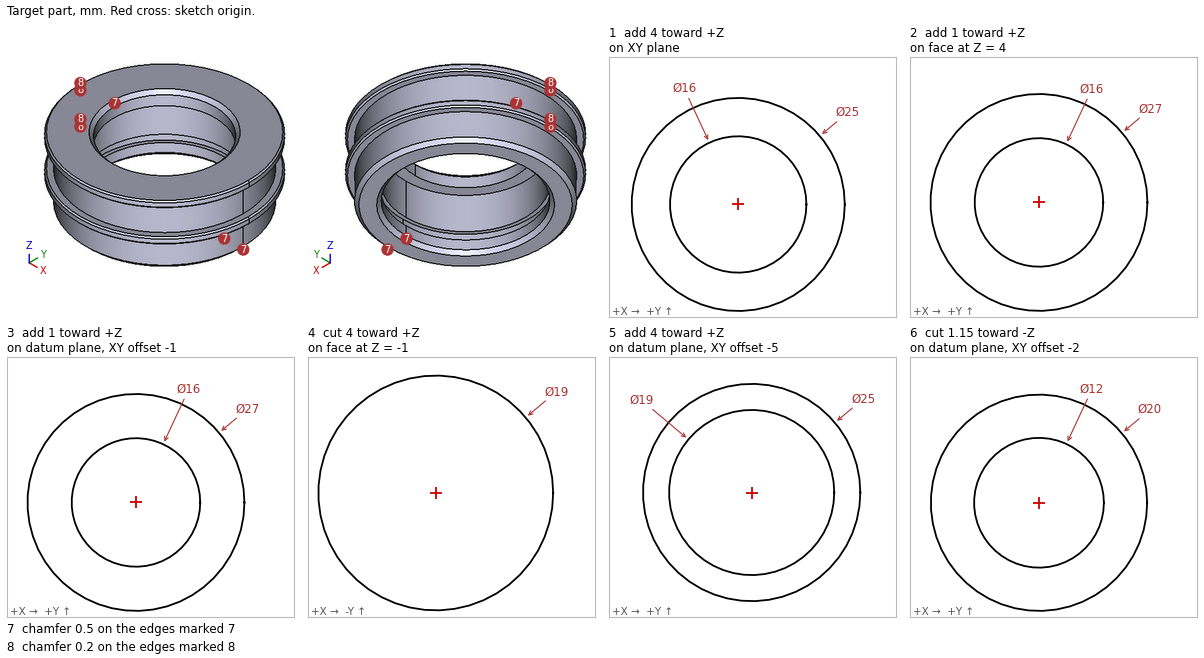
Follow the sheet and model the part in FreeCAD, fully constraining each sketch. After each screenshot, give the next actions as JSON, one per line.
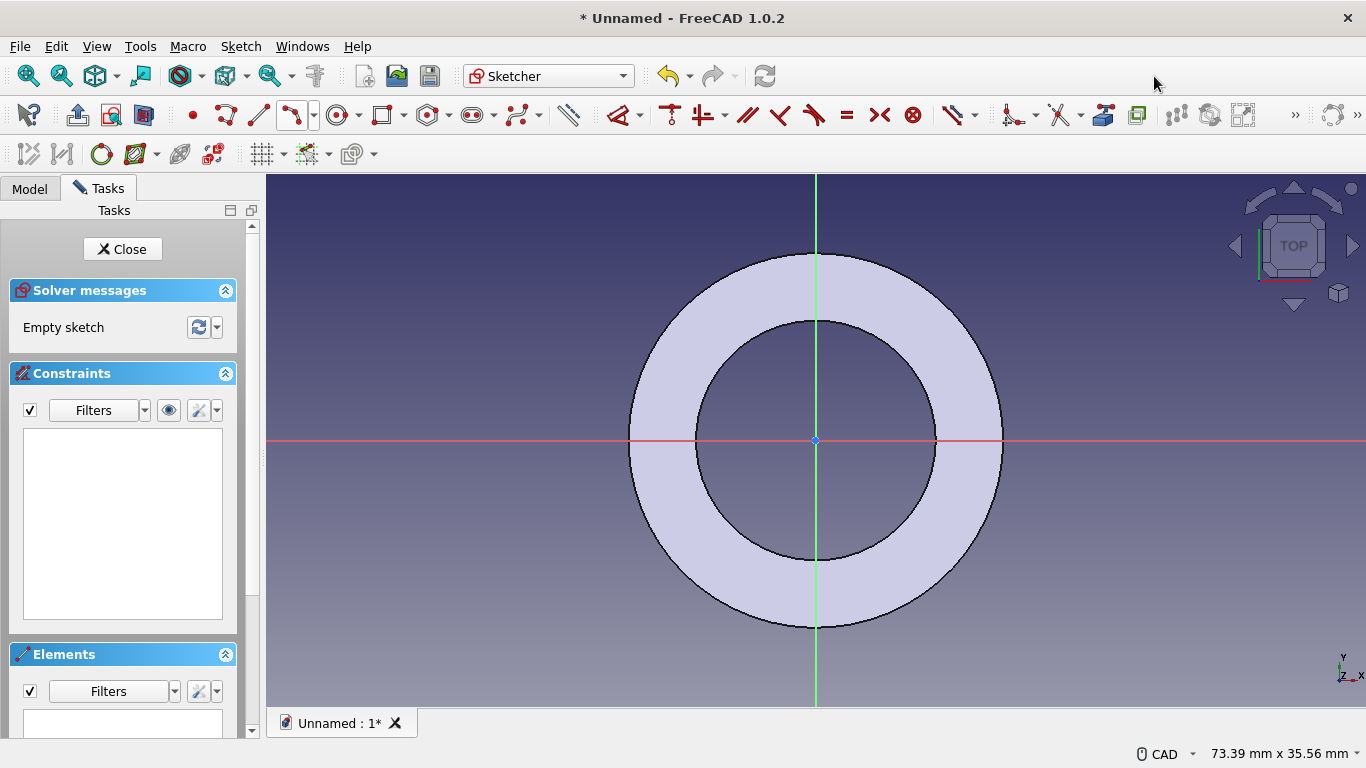
{"action": "left_click", "coordinate": [336, 116]}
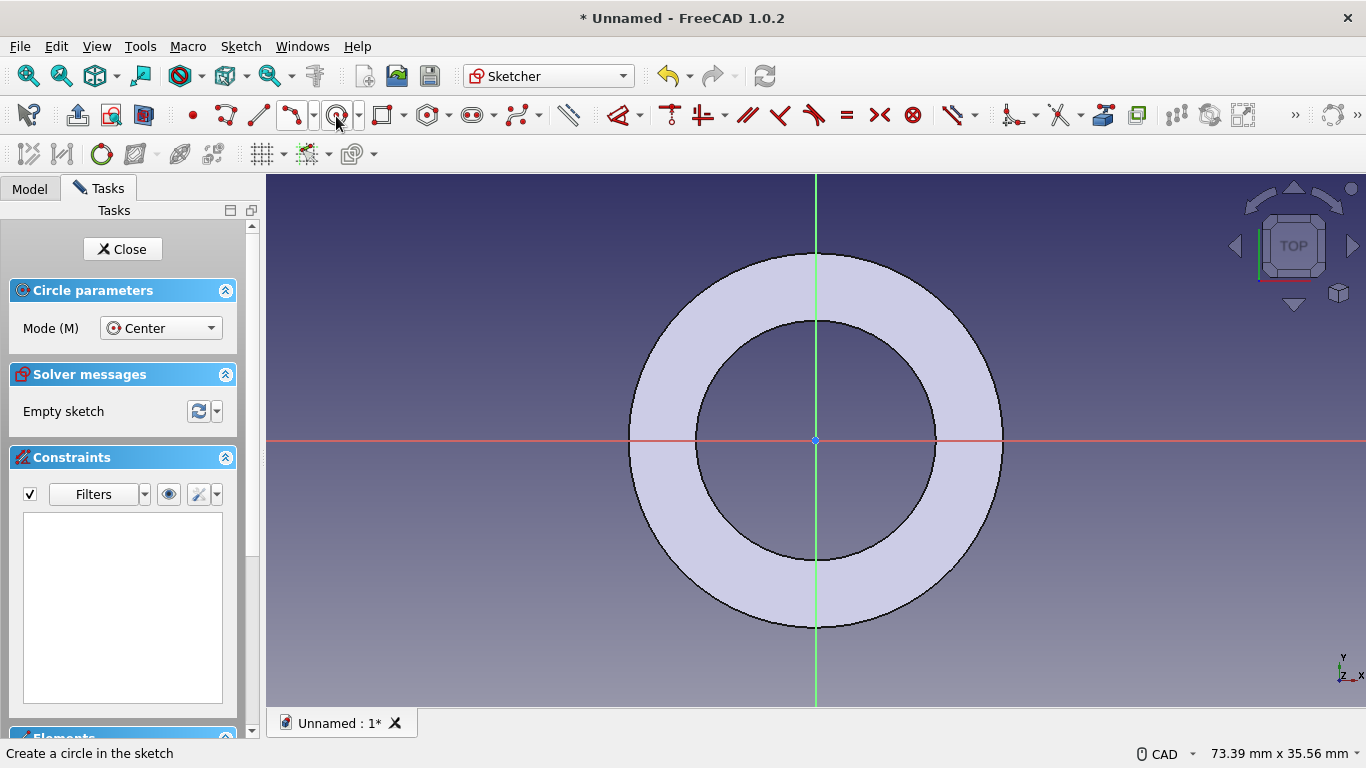
{"action": "left_click", "coordinate": [816, 440]}
{"action": "left_click", "coordinate": [959, 297]}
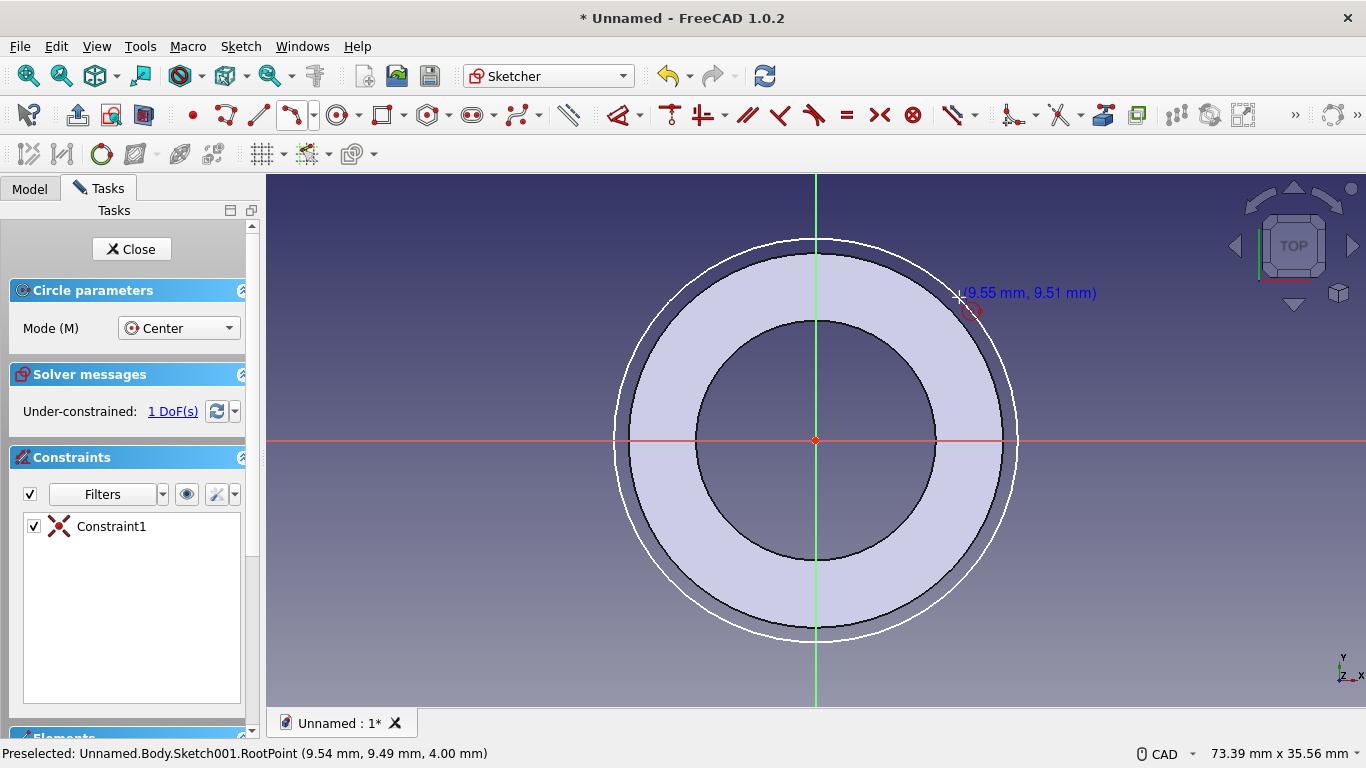
{"action": "left_click", "coordinate": [816, 440]}
{"action": "left_click", "coordinate": [901, 356]}
{"action": "key", "text": "Escape"}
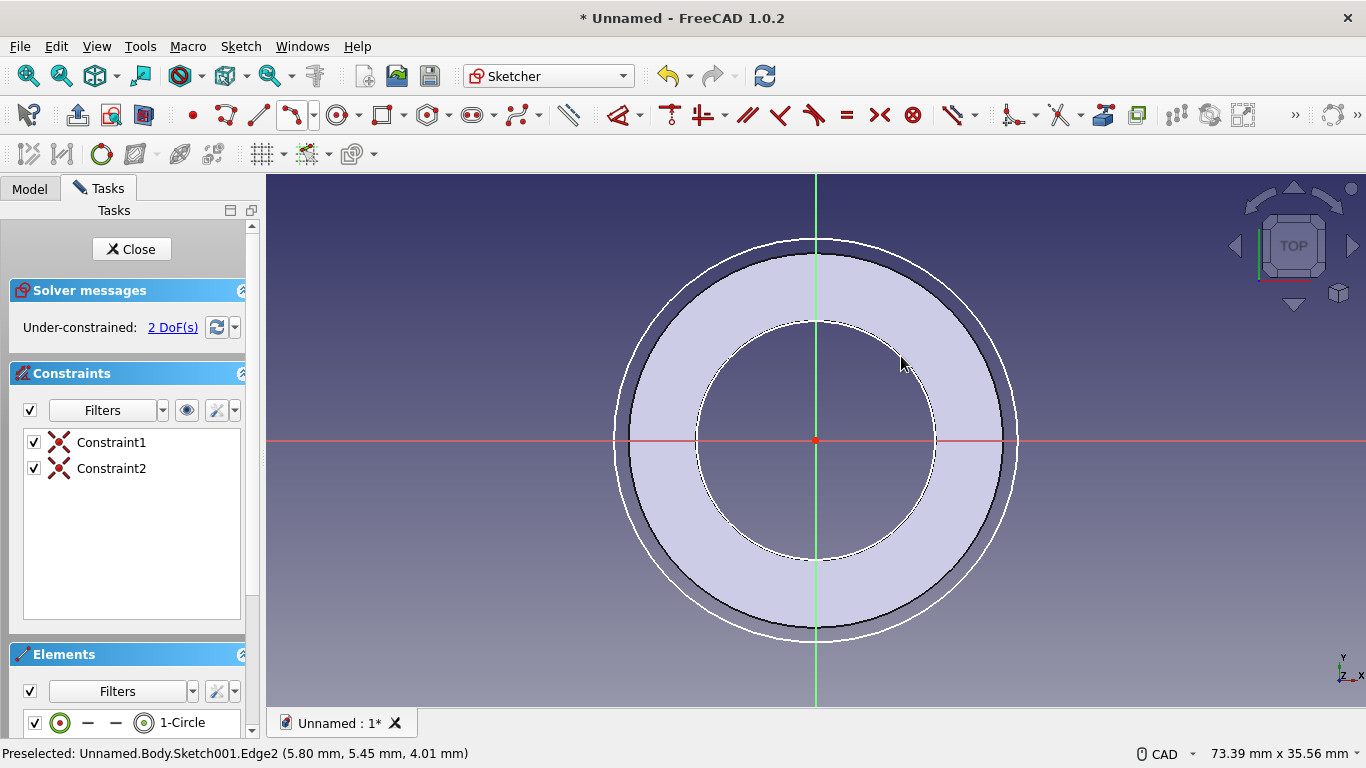
{"action": "left_click", "coordinate": [618, 116]}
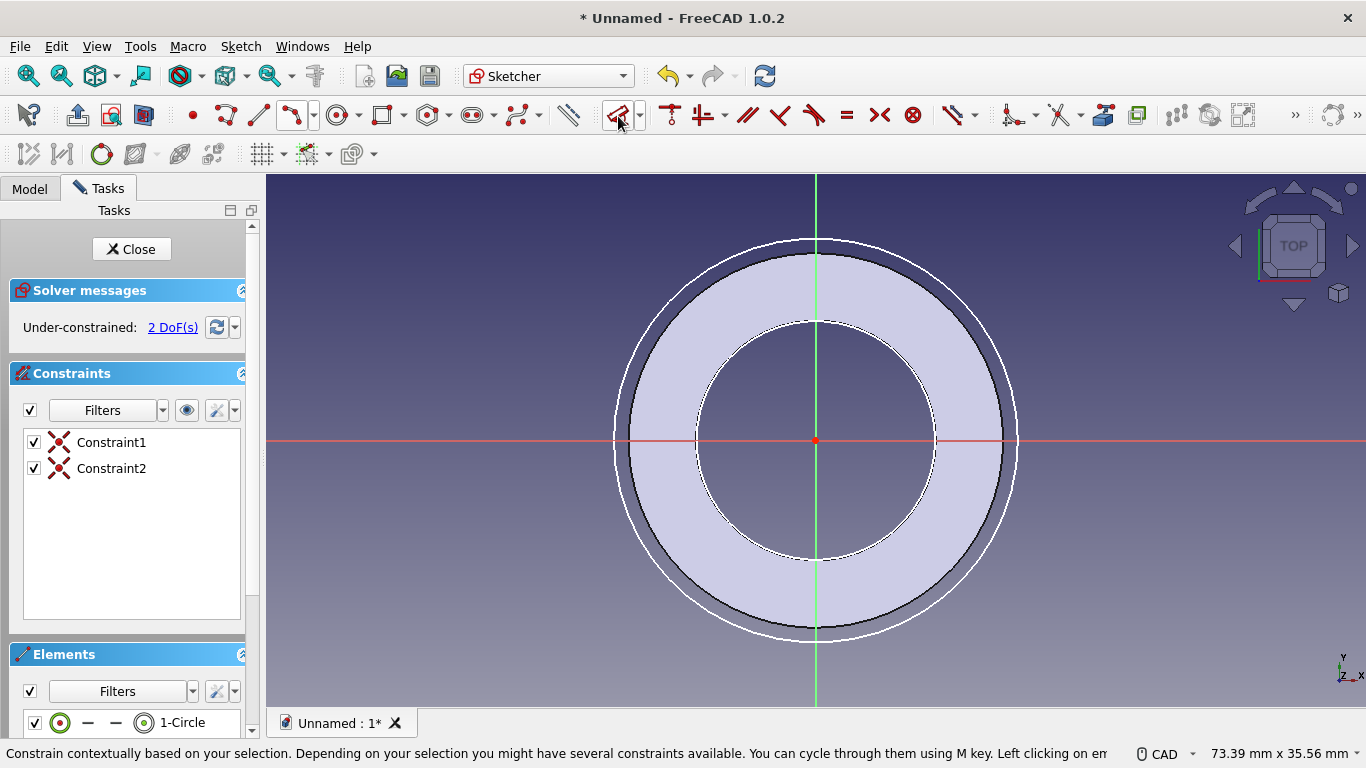
{"action": "left_click", "coordinate": [958, 297]}
{"action": "left_click", "coordinate": [981, 274]}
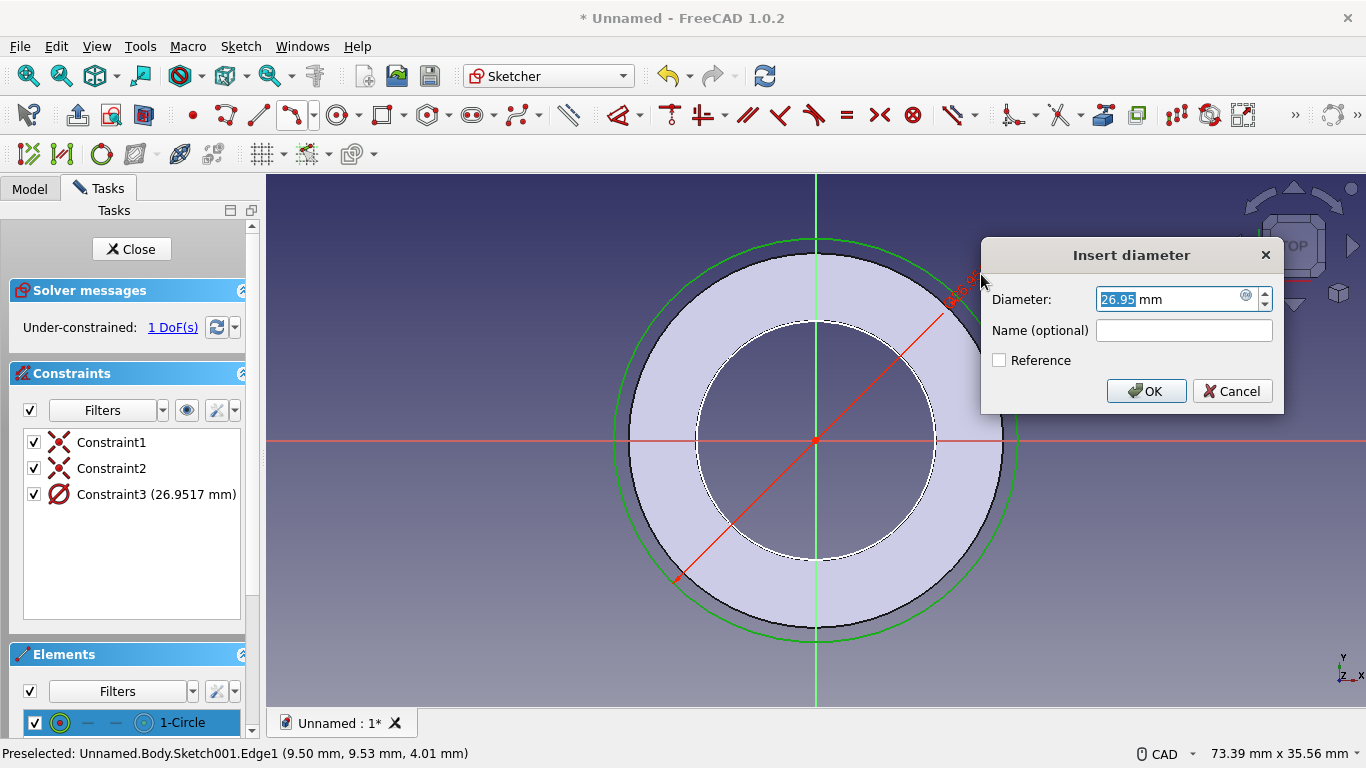
{"action": "type", "text": "27"}
{"action": "key", "text": "Return"}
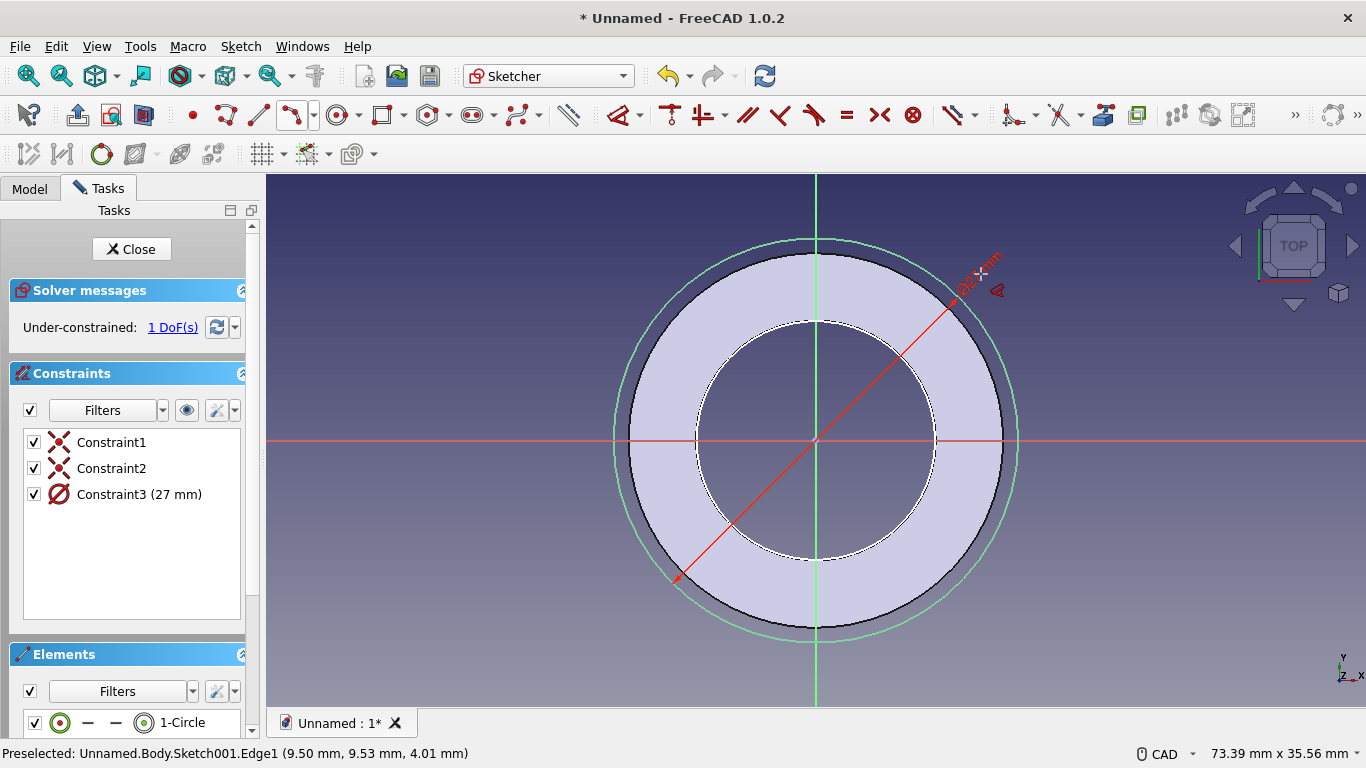
{"action": "left_click", "coordinate": [900, 356]}
{"action": "left_click", "coordinate": [923, 333]}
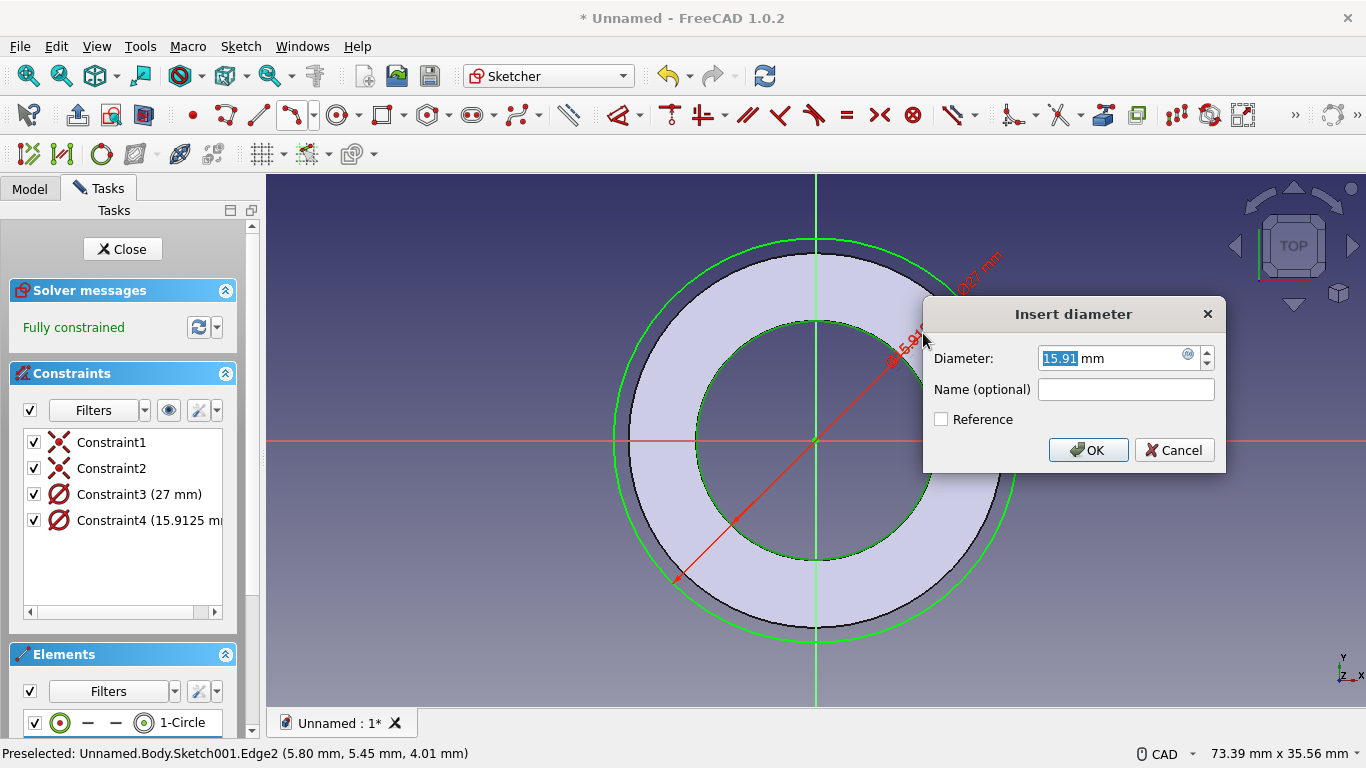
{"action": "type", "text": "16"}
{"action": "key", "text": "Return"}
{"action": "key", "text": "Escape"}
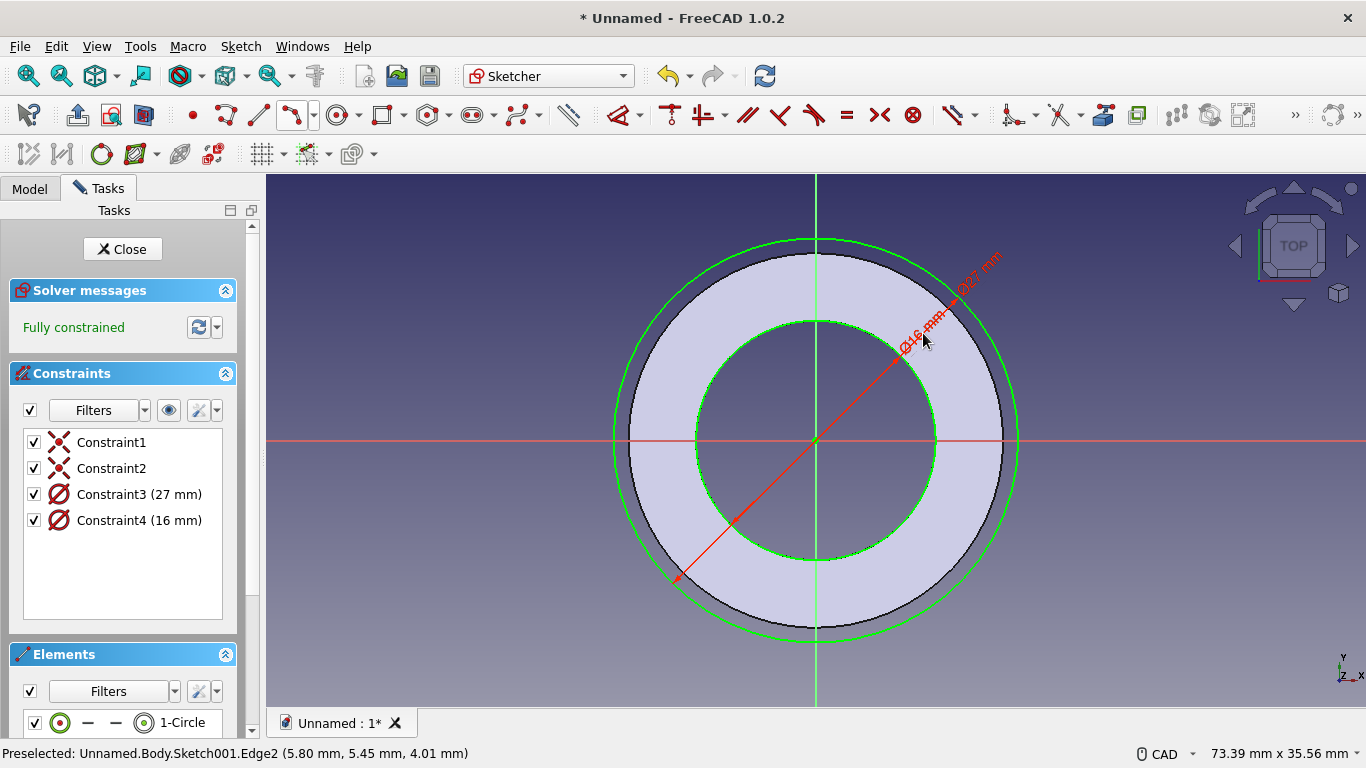
{"action": "left_click", "coordinate": [123, 249]}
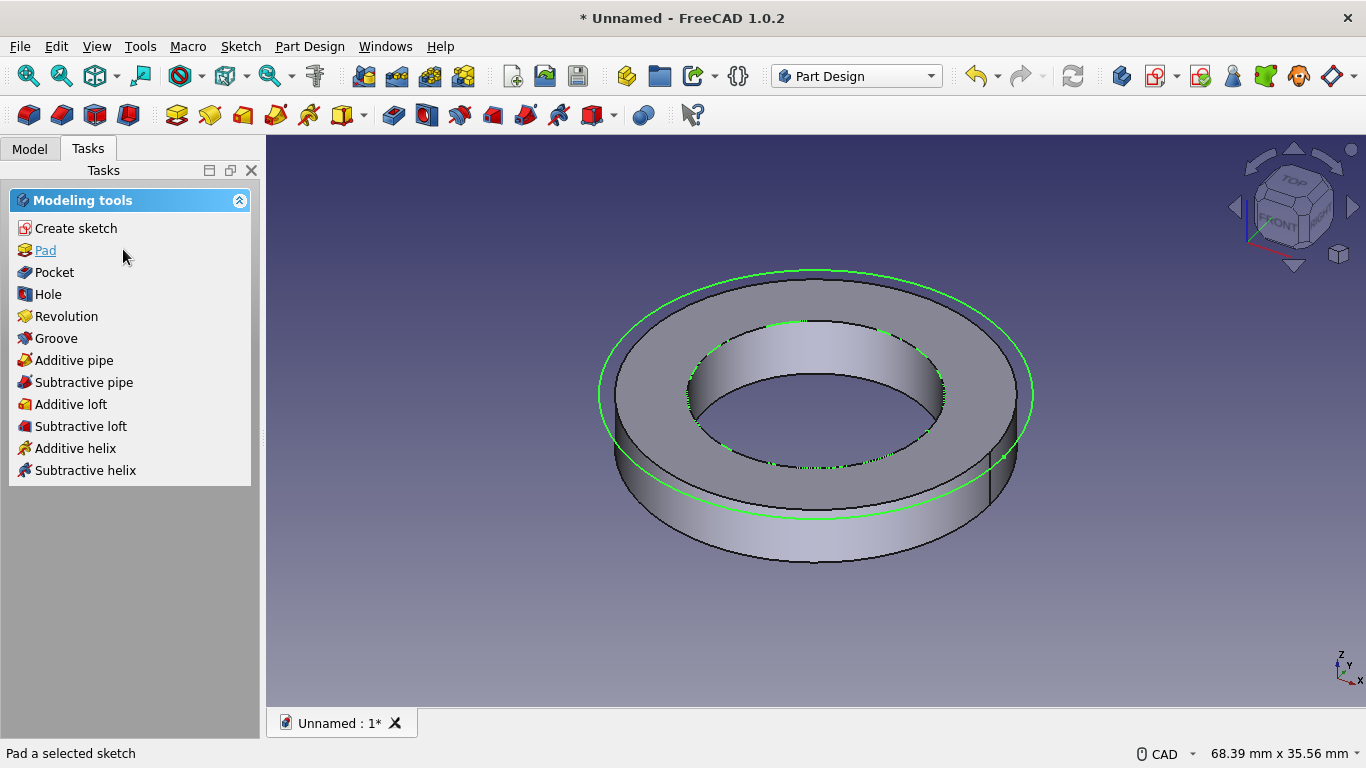
{"action": "left_click", "coordinate": [177, 116]}